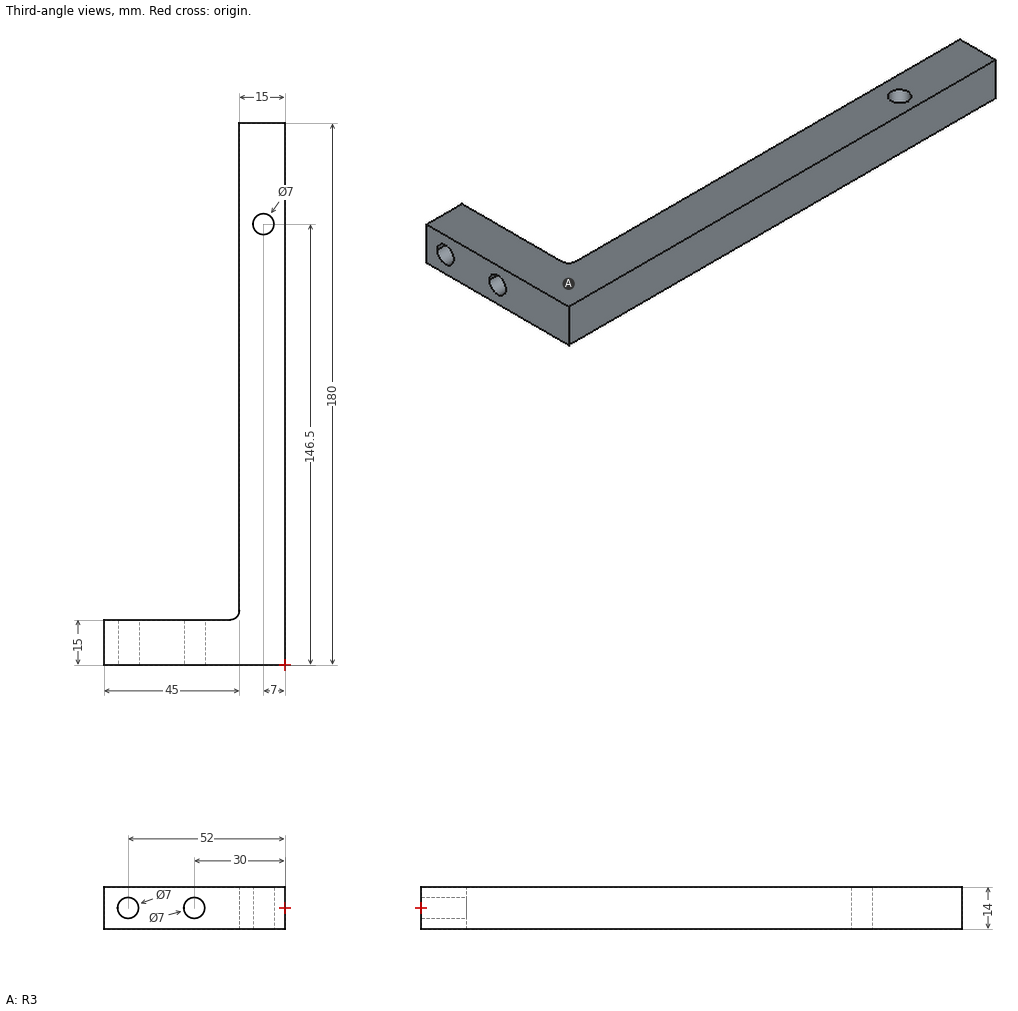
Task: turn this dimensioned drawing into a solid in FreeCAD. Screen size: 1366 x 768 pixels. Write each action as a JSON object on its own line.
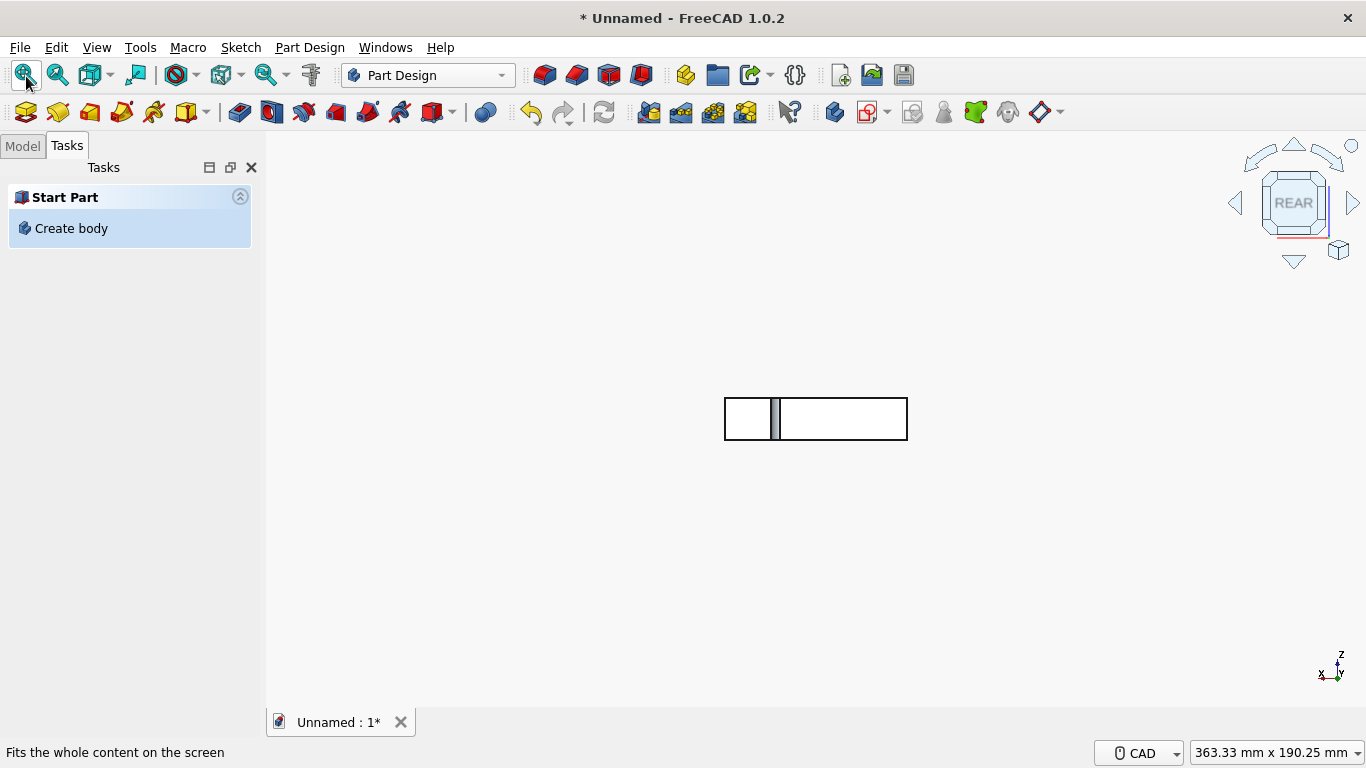
{"action": "left_click", "coordinate": [807, 418]}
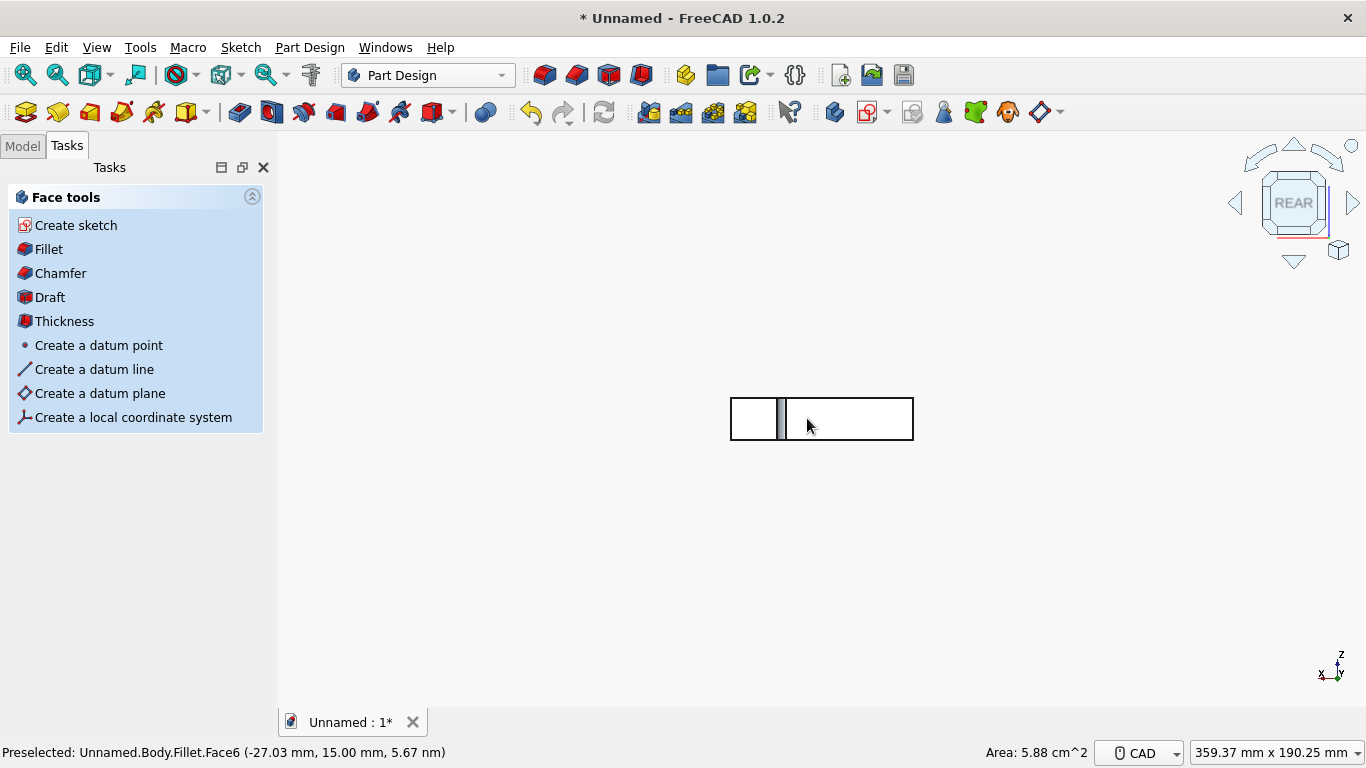
{"action": "left_click", "coordinate": [868, 112]}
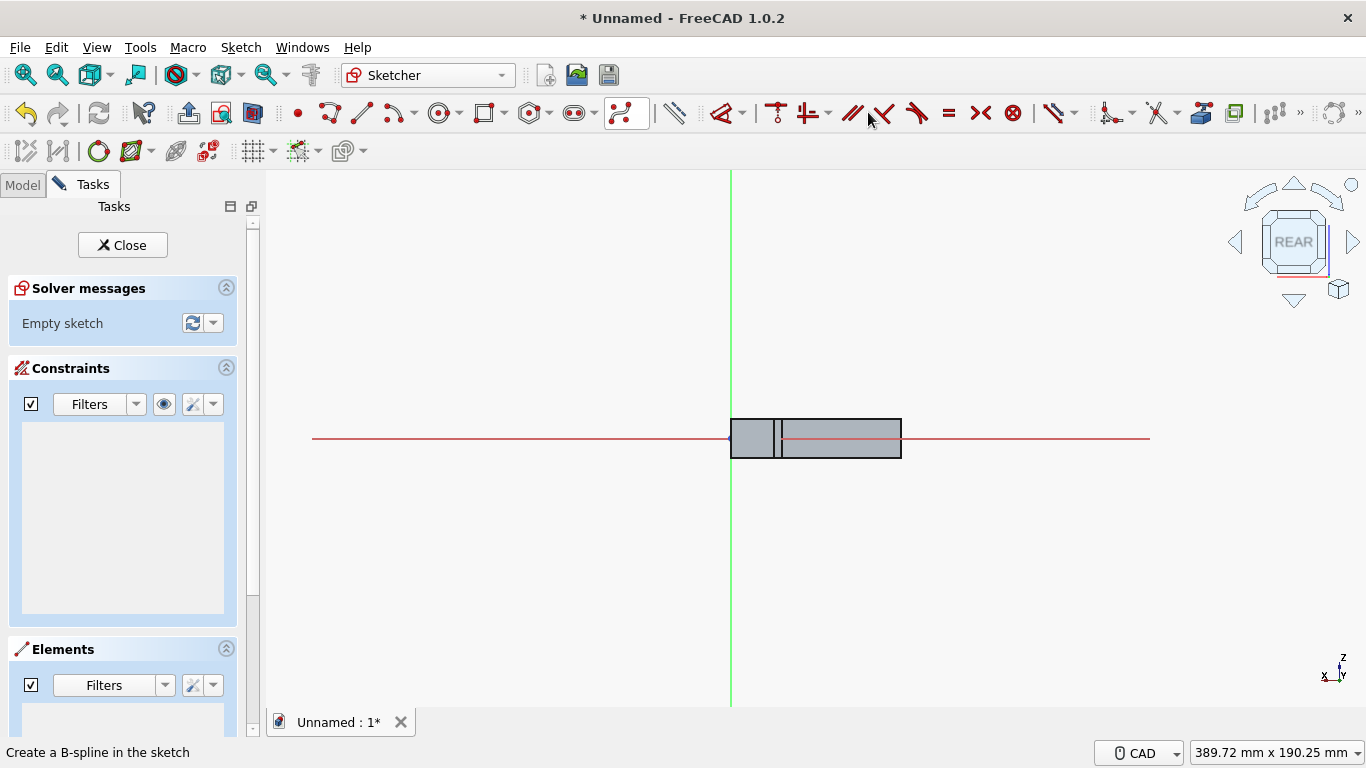
{"action": "left_click", "coordinate": [254, 114]}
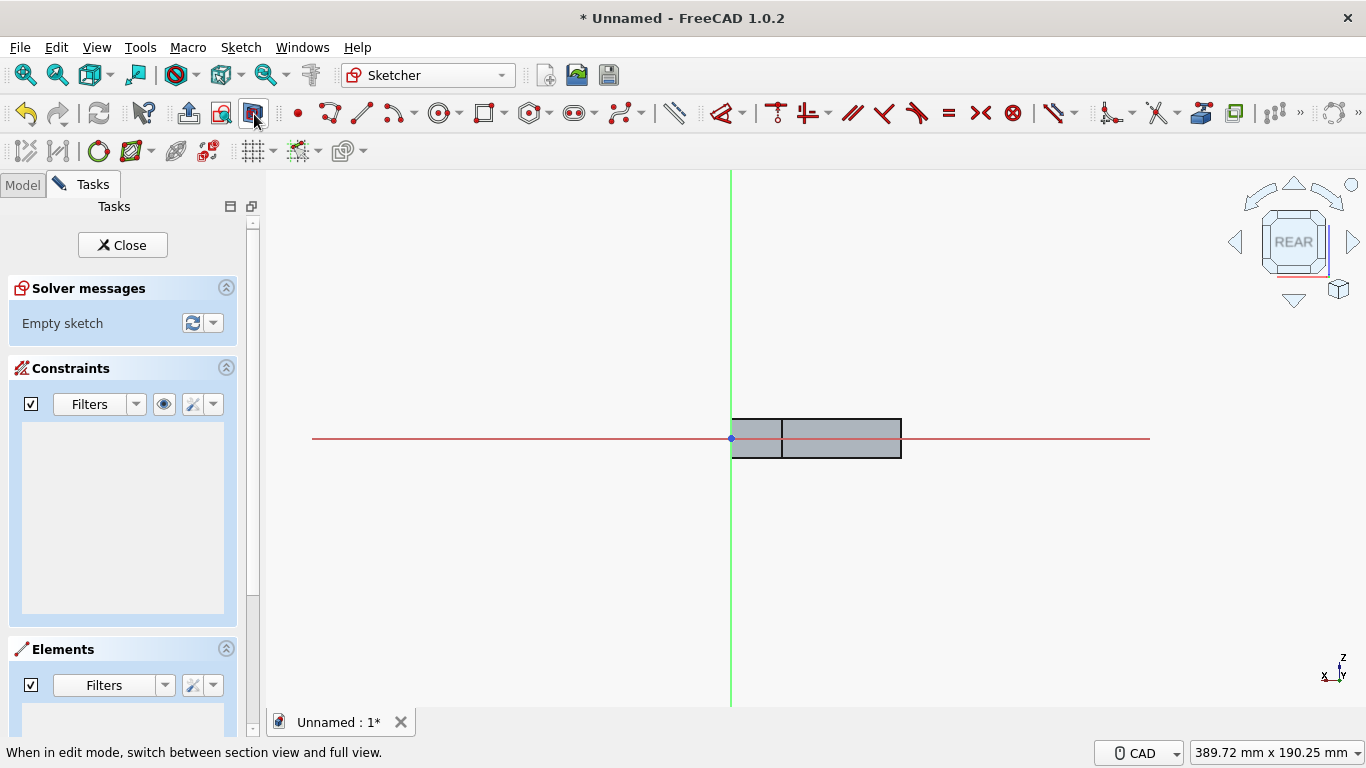
{"action": "scroll", "coordinate": [887, 439], "scroll_direction": "up", "scroll_amount": 14}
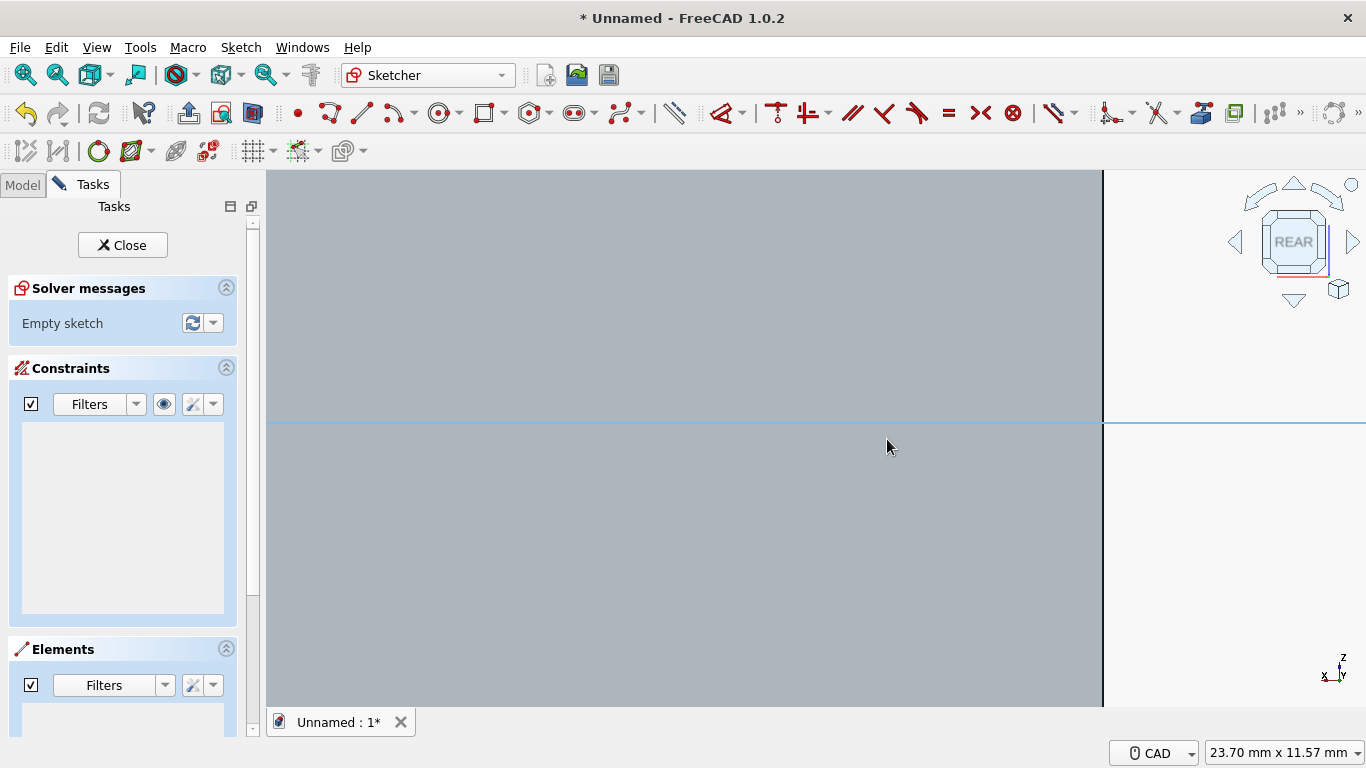
{"action": "left_click", "coordinate": [440, 114]}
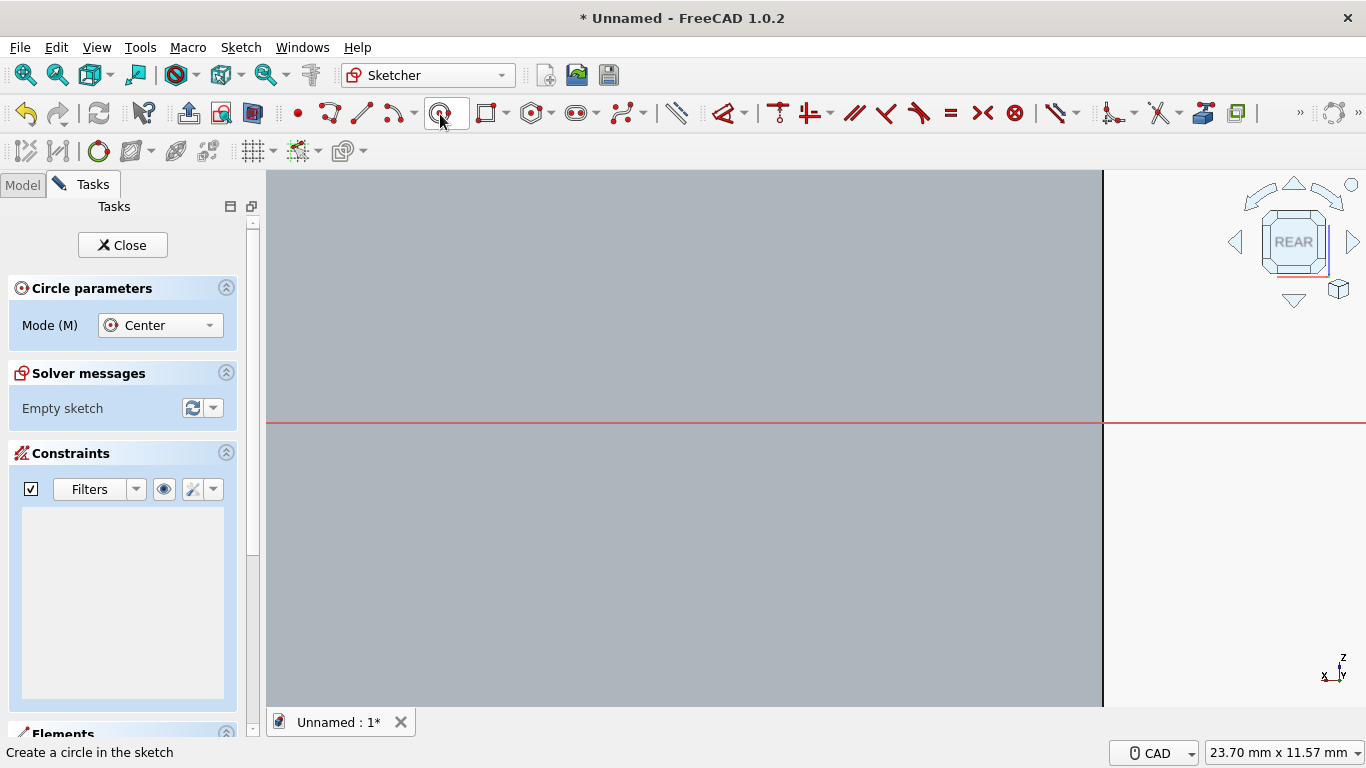
{"action": "left_click", "coordinate": [732, 423]}
{"action": "mouse_move", "coordinate": [847, 308]}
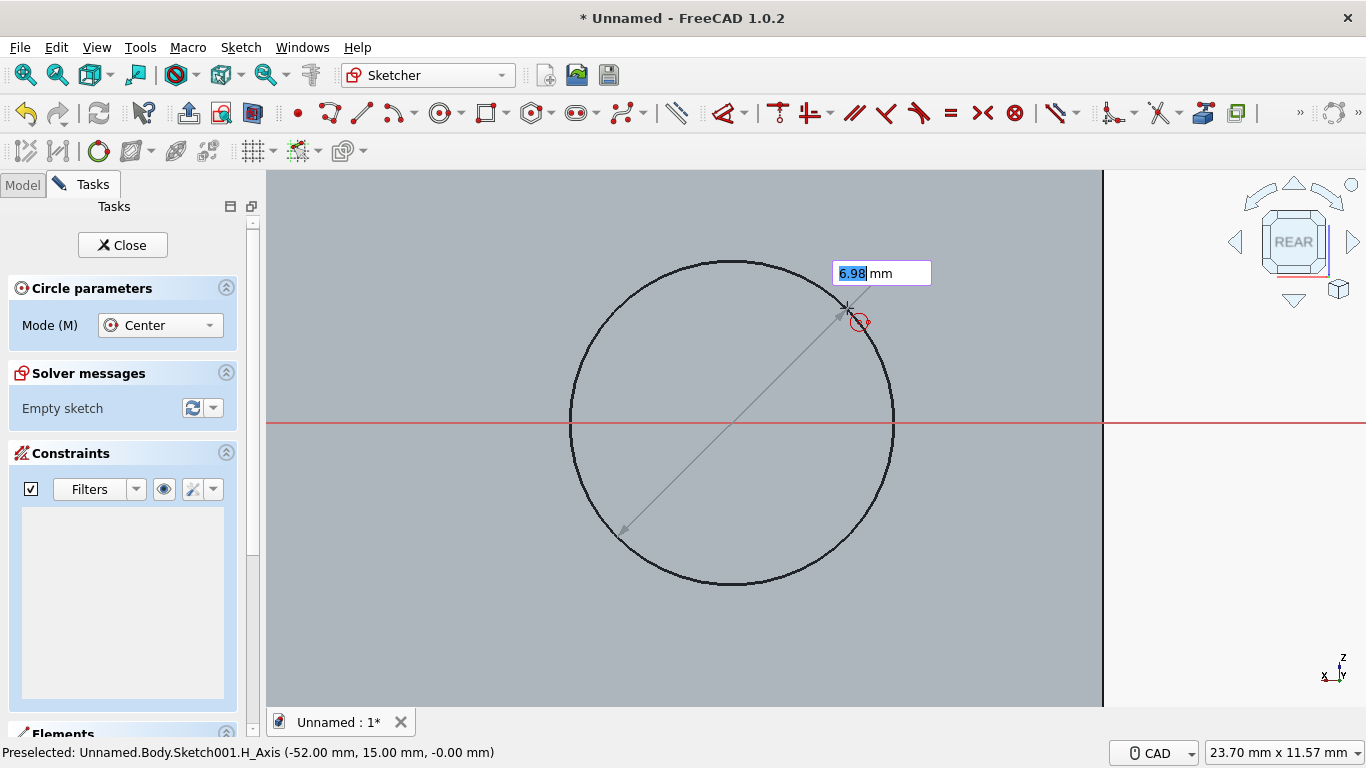
{"action": "type", "text": "7"}
{"action": "key", "text": "Return"}
{"action": "key", "text": "Escape"}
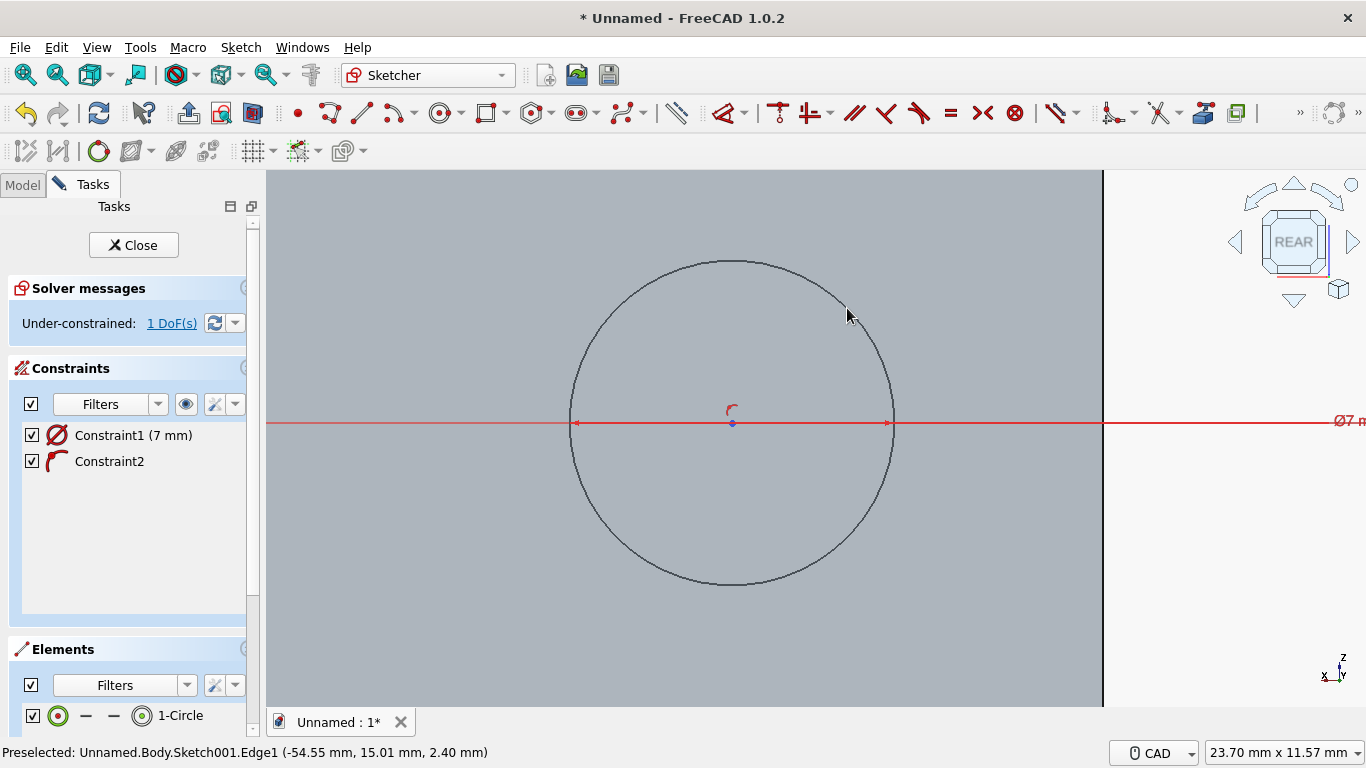
{"action": "left_click", "coordinate": [724, 114]}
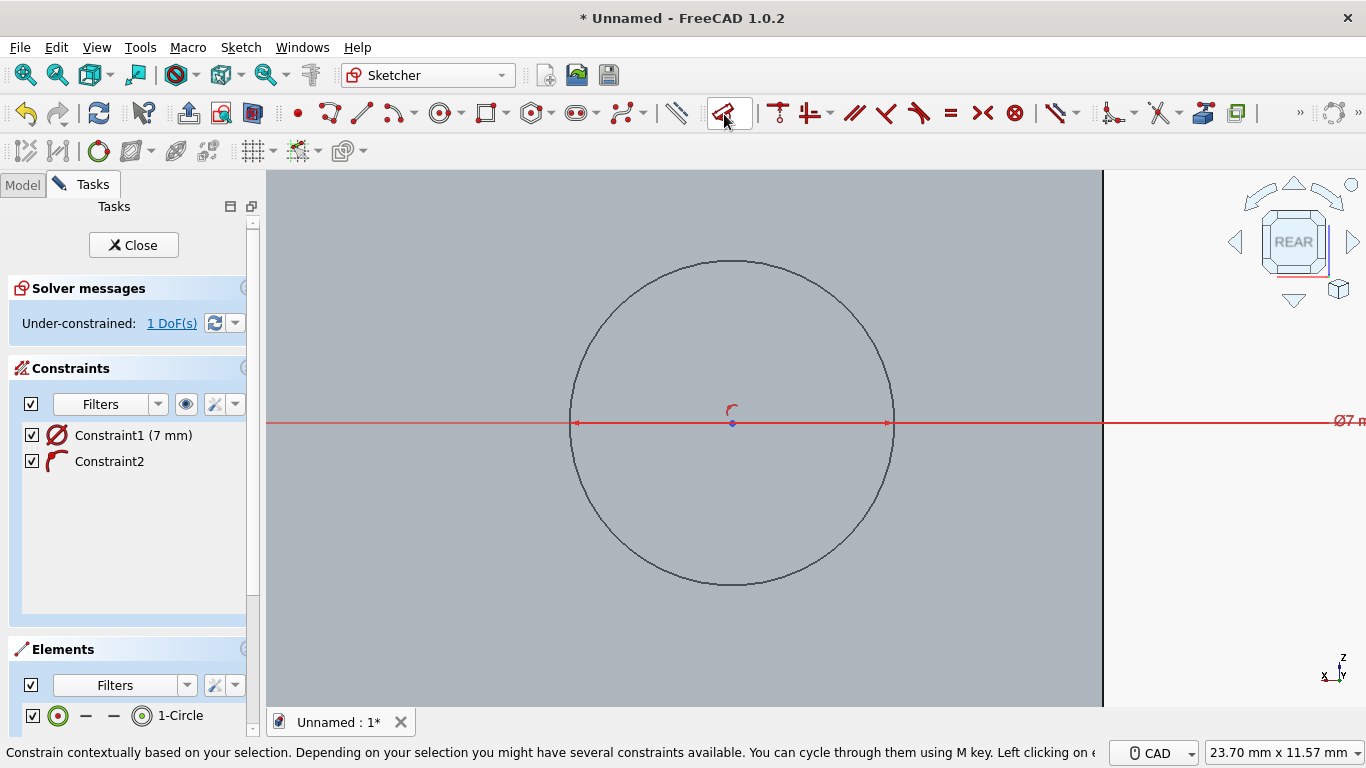
{"action": "left_click", "coordinate": [732, 423]}
{"action": "left_click", "coordinate": [513, 457]}